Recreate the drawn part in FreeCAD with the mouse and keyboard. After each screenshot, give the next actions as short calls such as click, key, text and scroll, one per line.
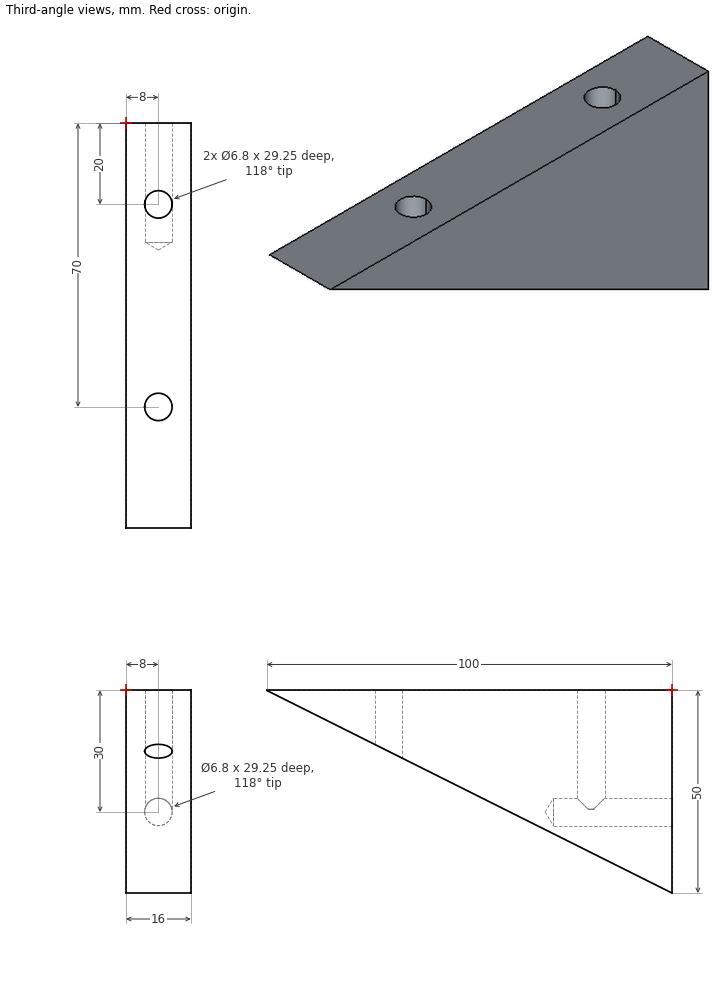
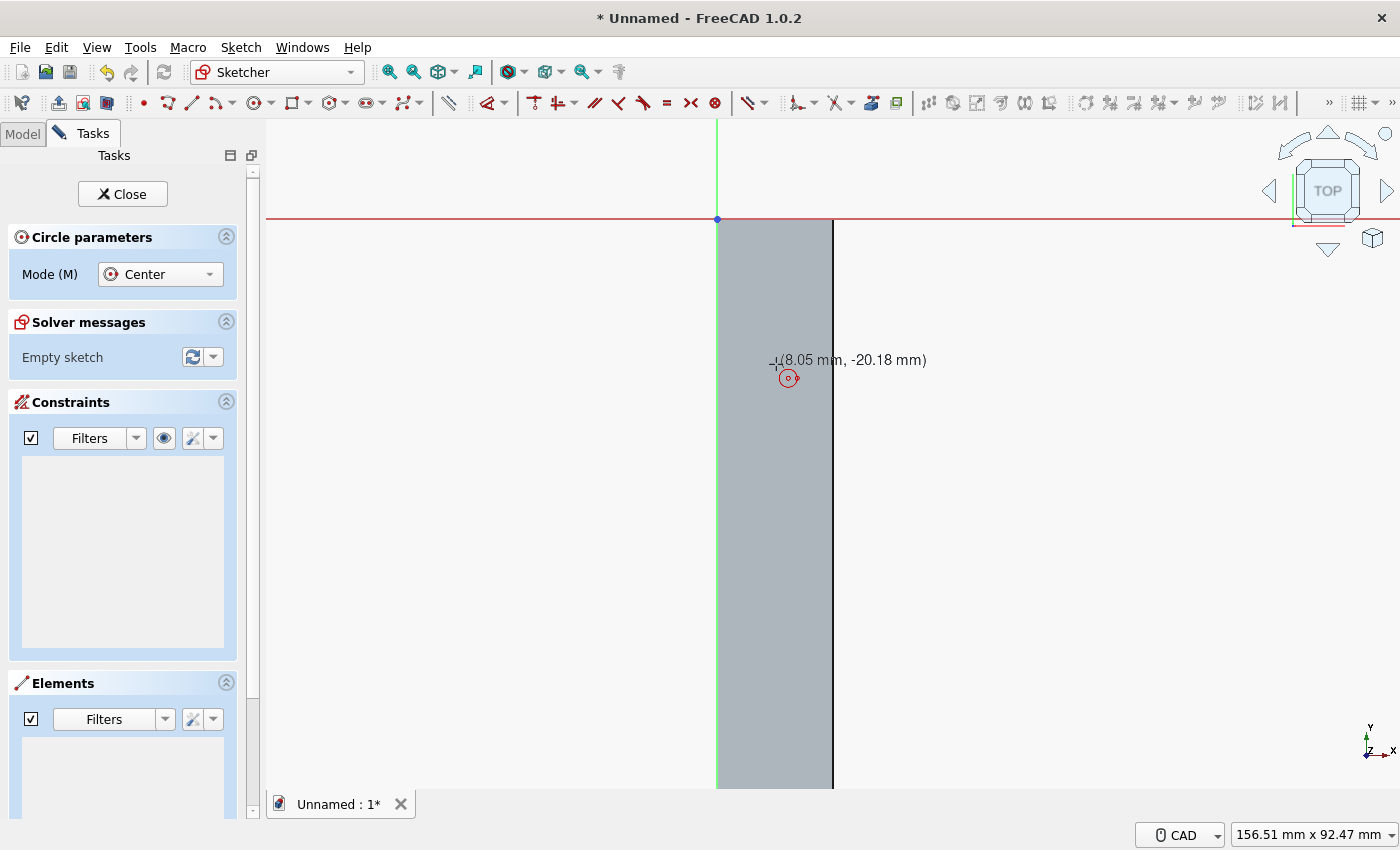
click(775, 364)
click(793, 347)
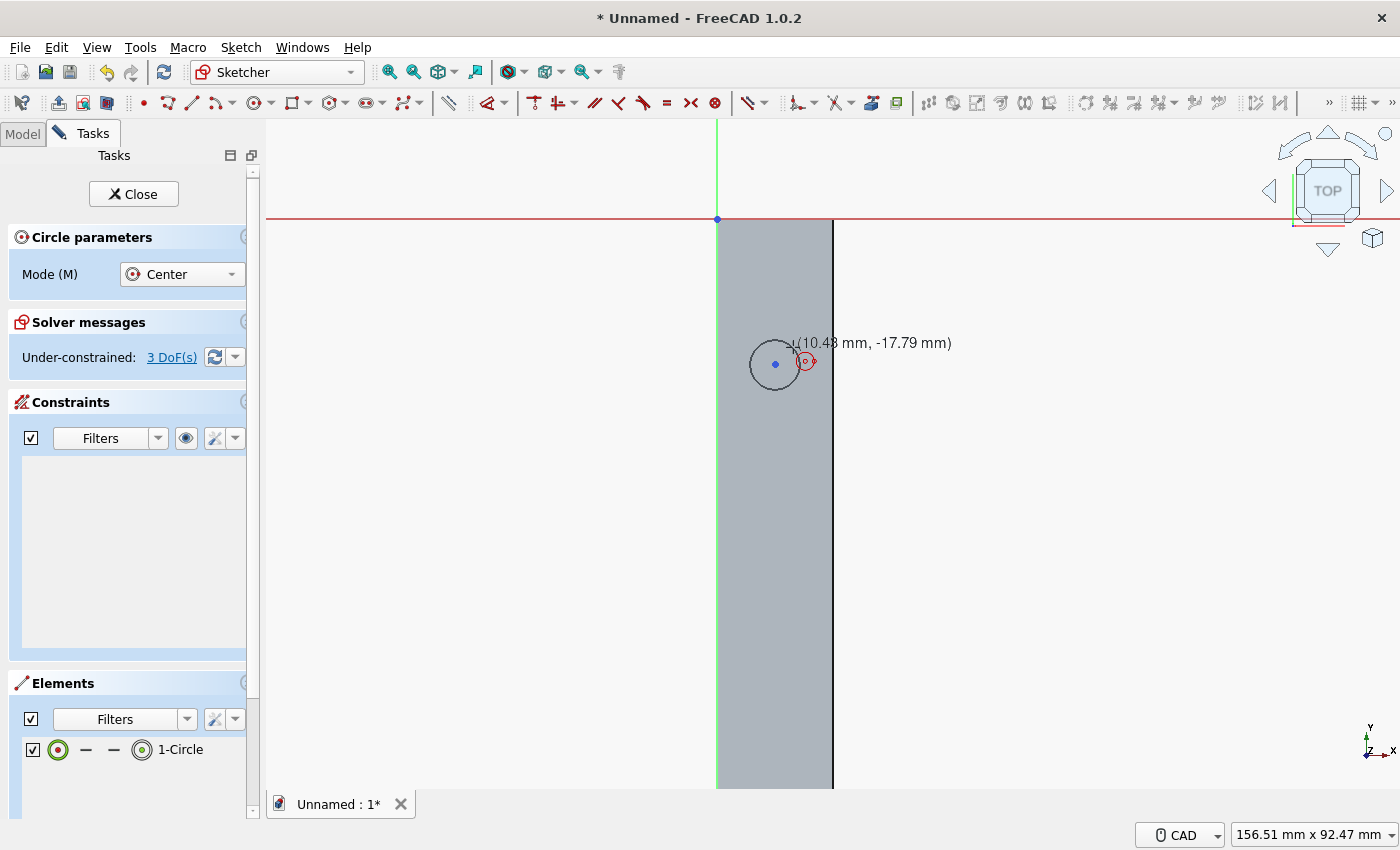
click(775, 726)
click(793, 709)
key(Escape)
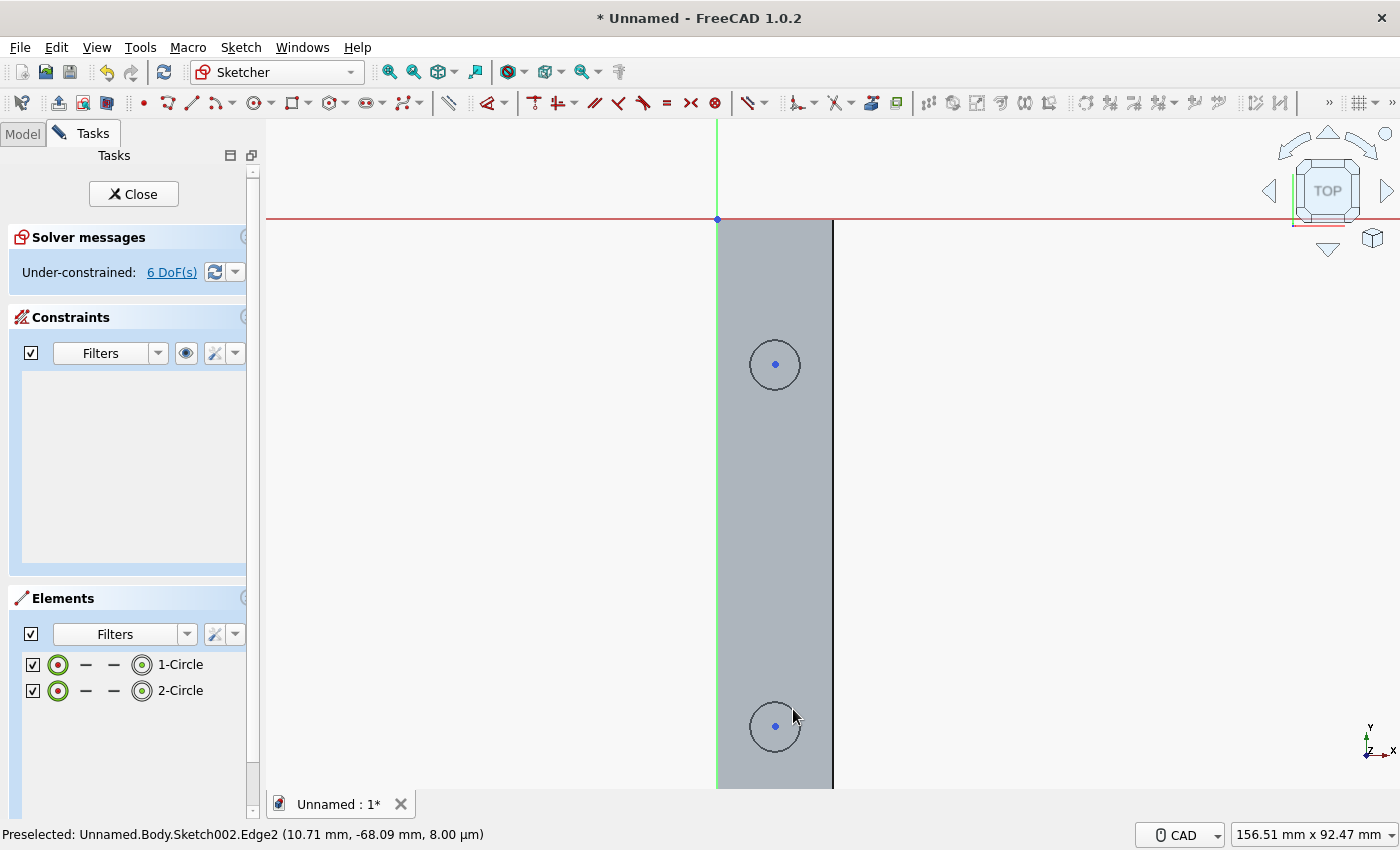
click(792, 347)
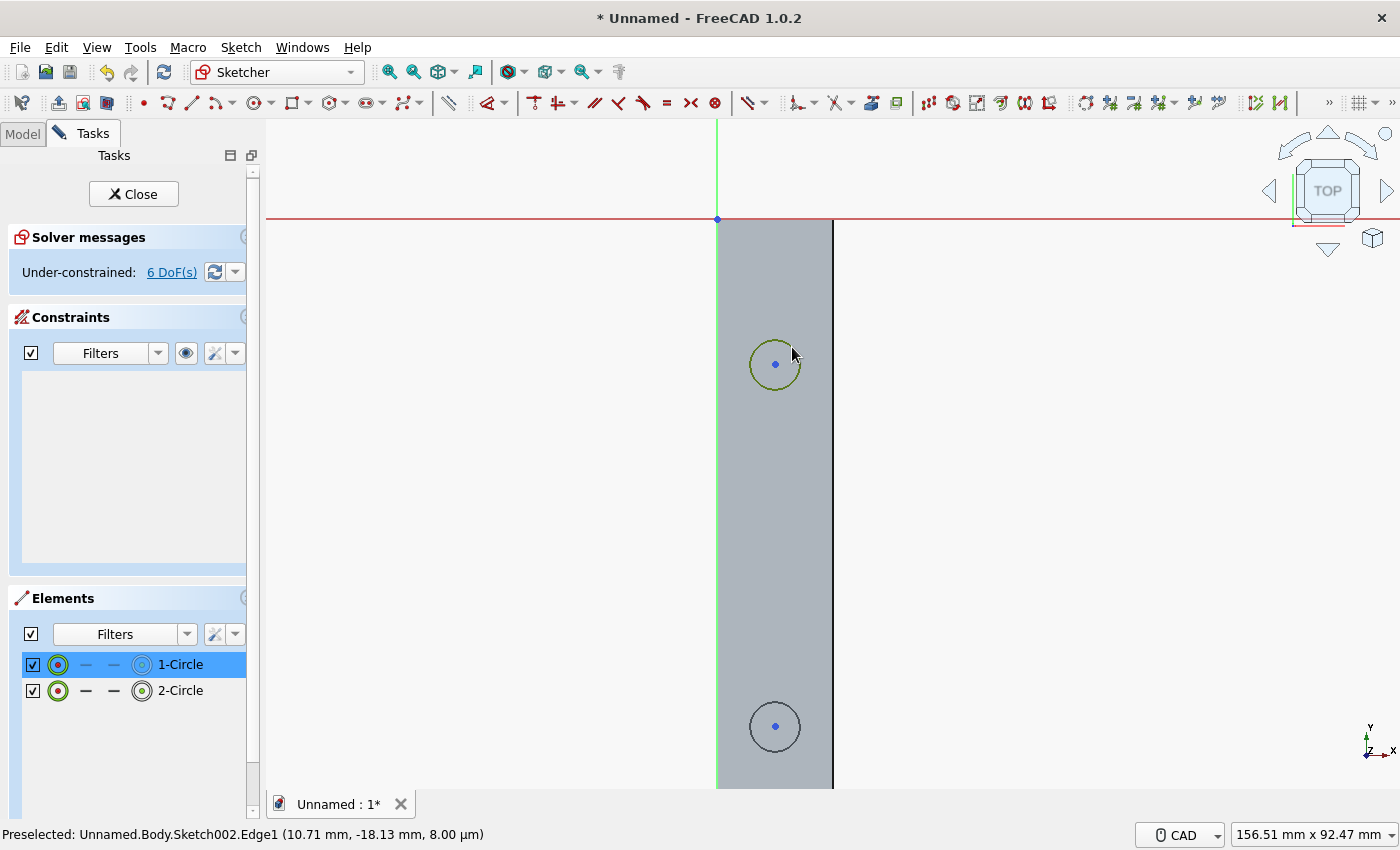
click(792, 709)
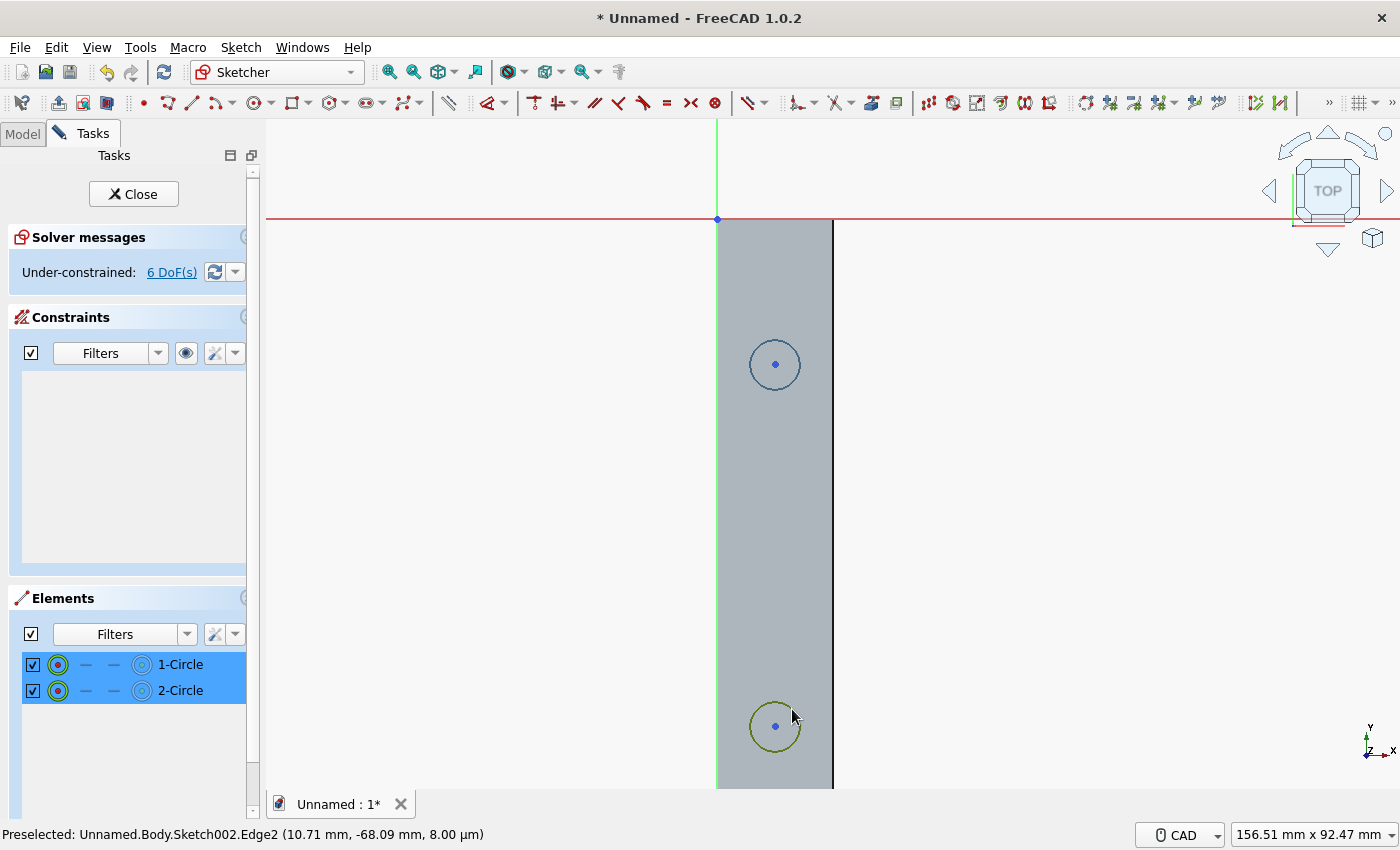
click(668, 104)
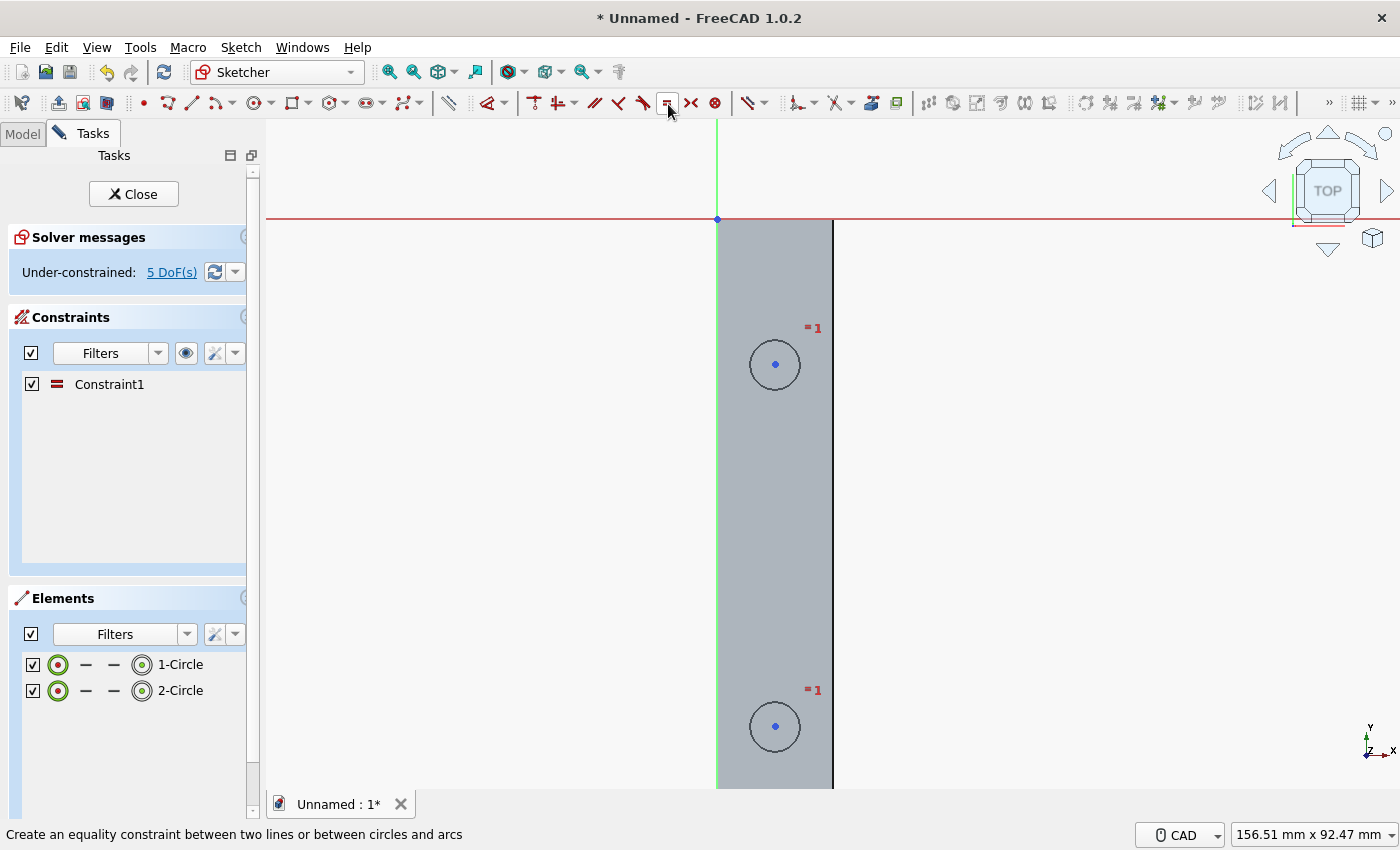
click(775, 365)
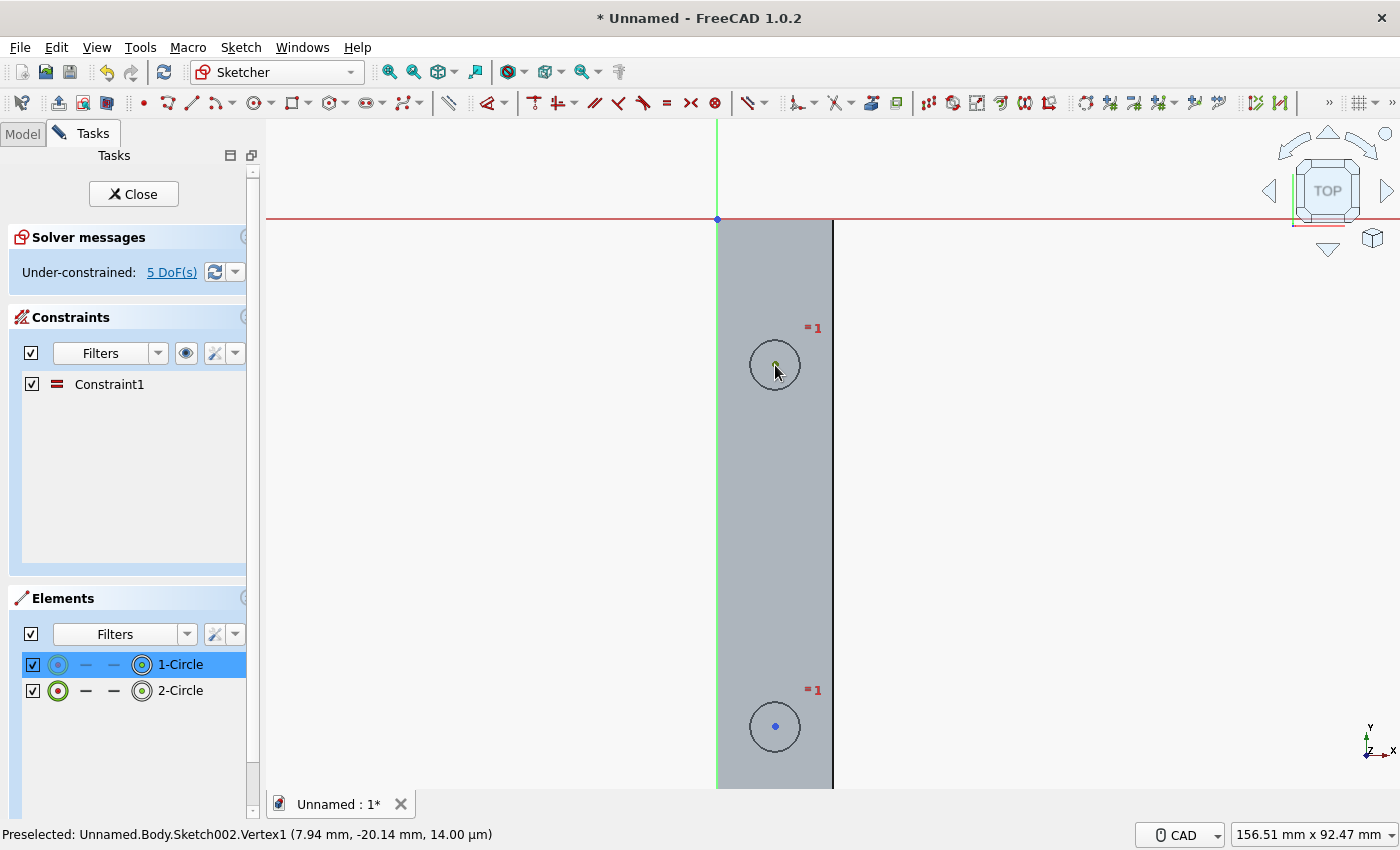
click(775, 727)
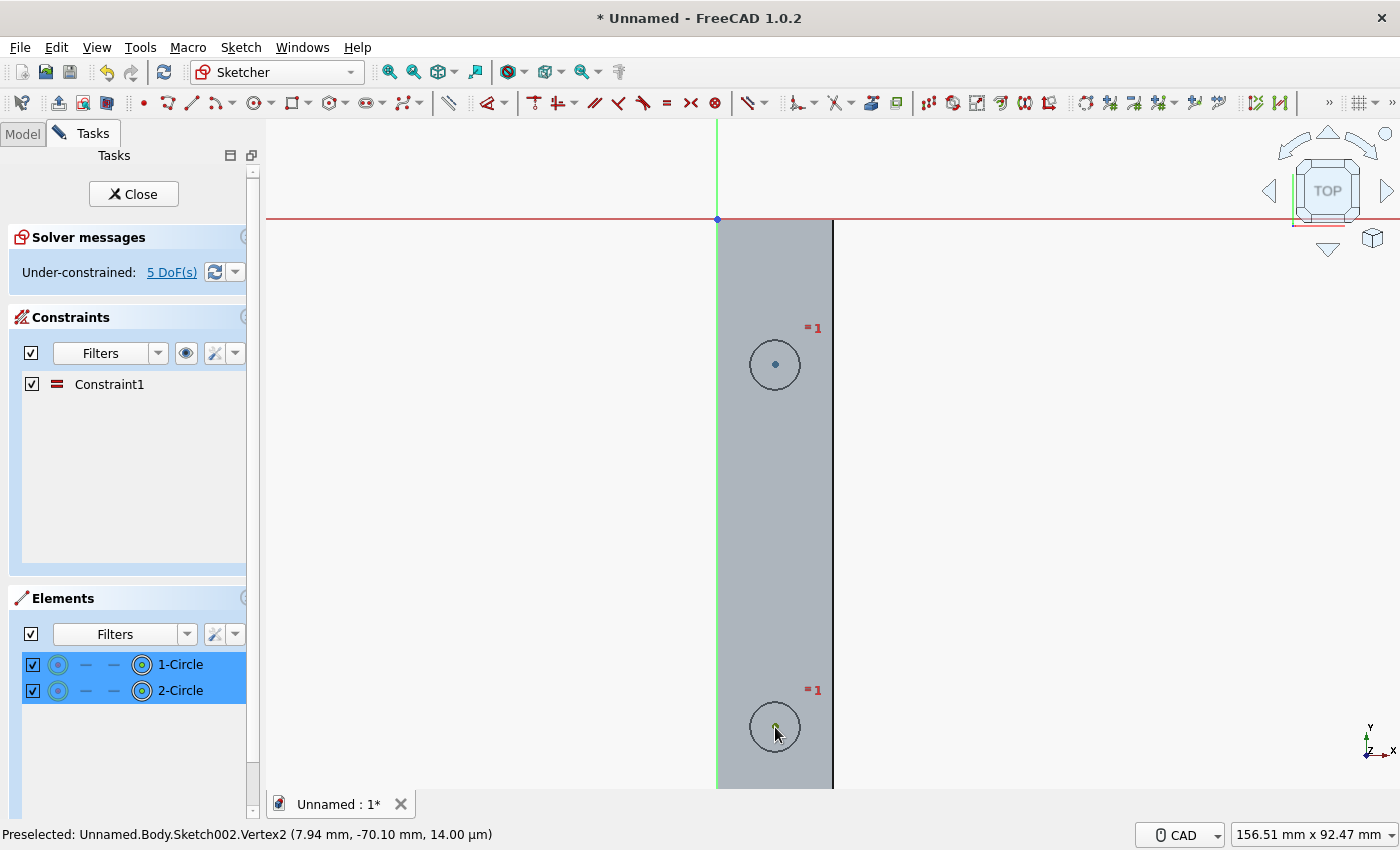
click(576, 104)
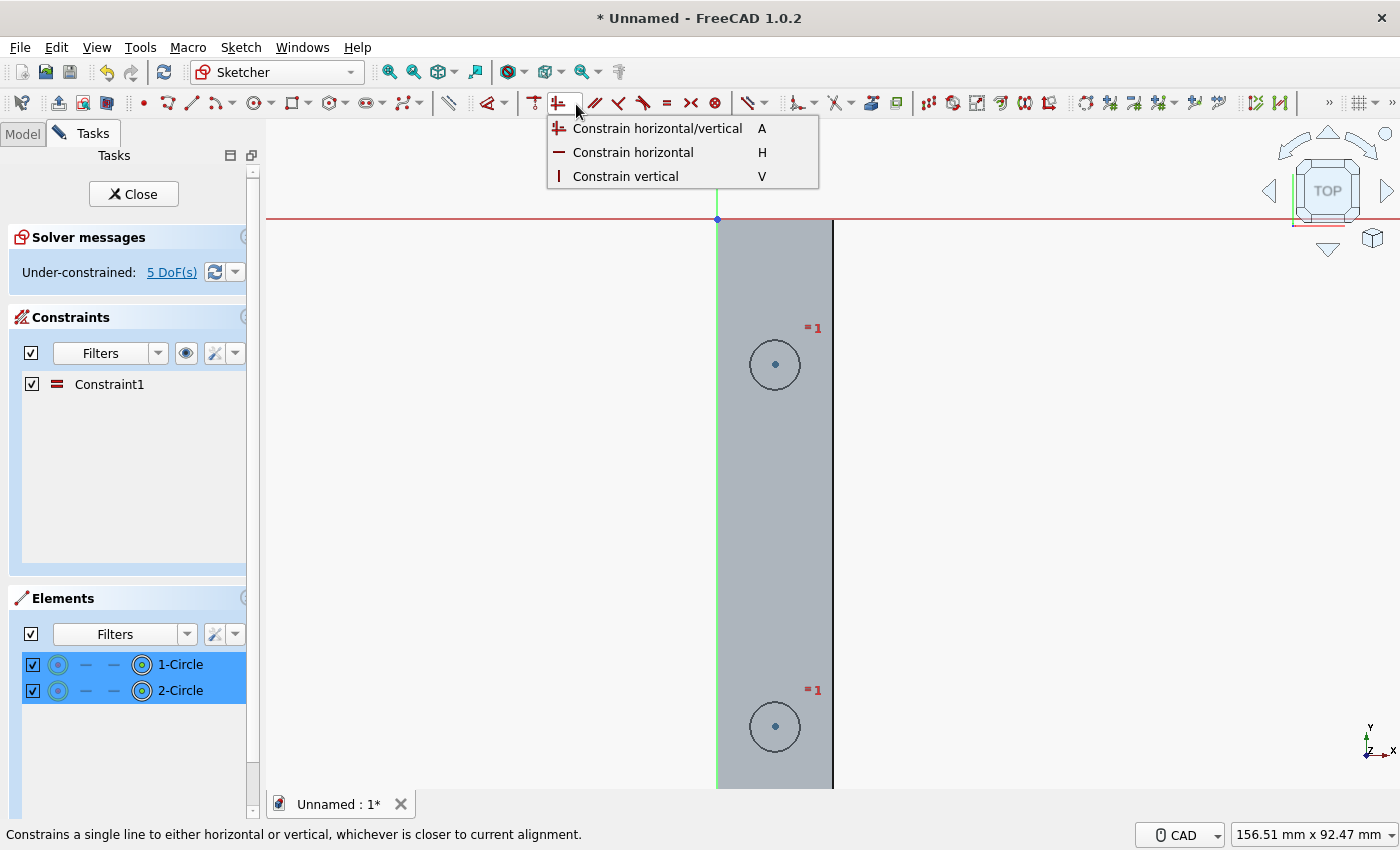
click(683, 176)